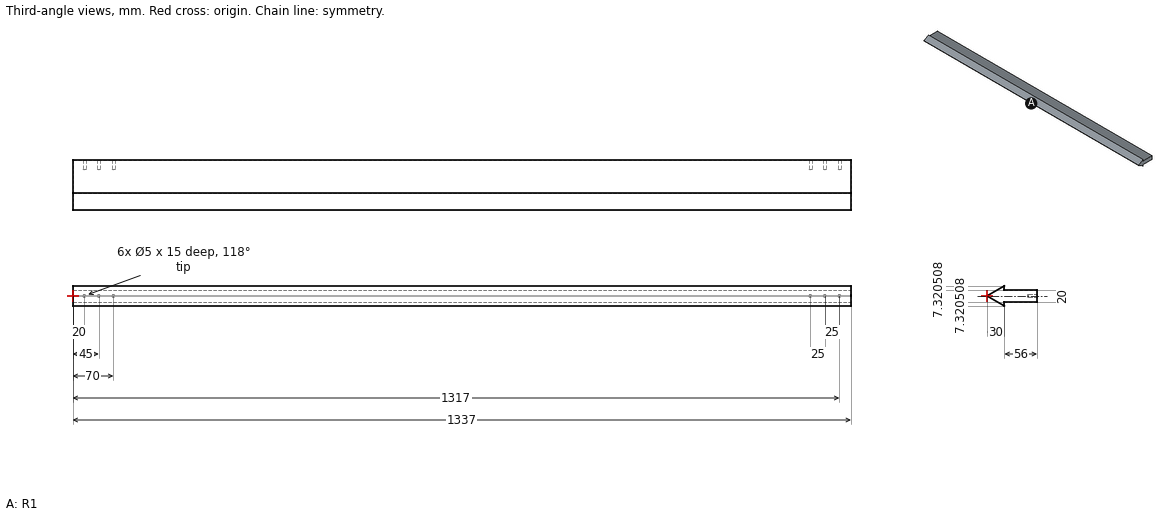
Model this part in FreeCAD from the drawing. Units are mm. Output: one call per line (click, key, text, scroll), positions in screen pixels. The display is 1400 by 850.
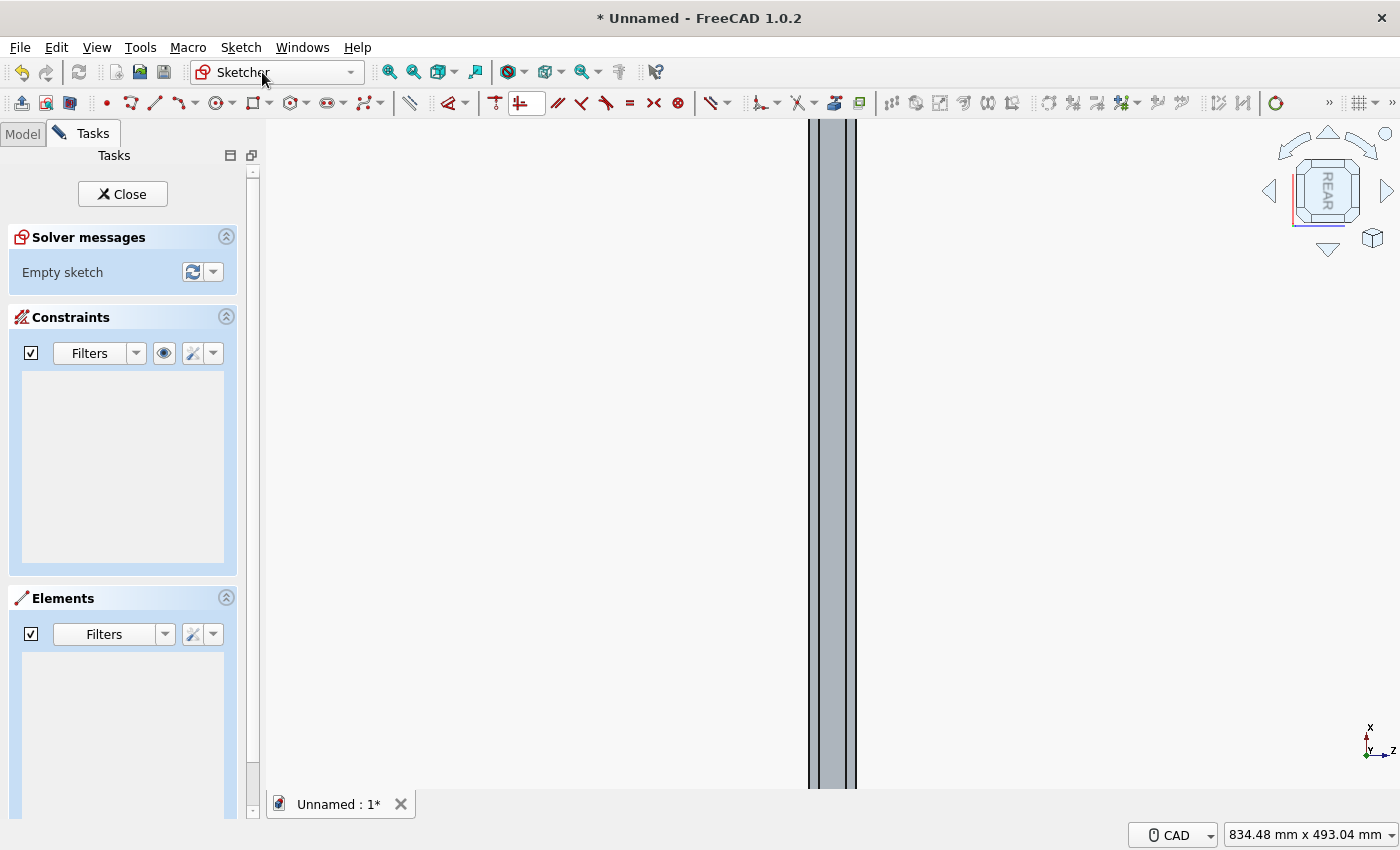
scroll(742, 450, down, 7)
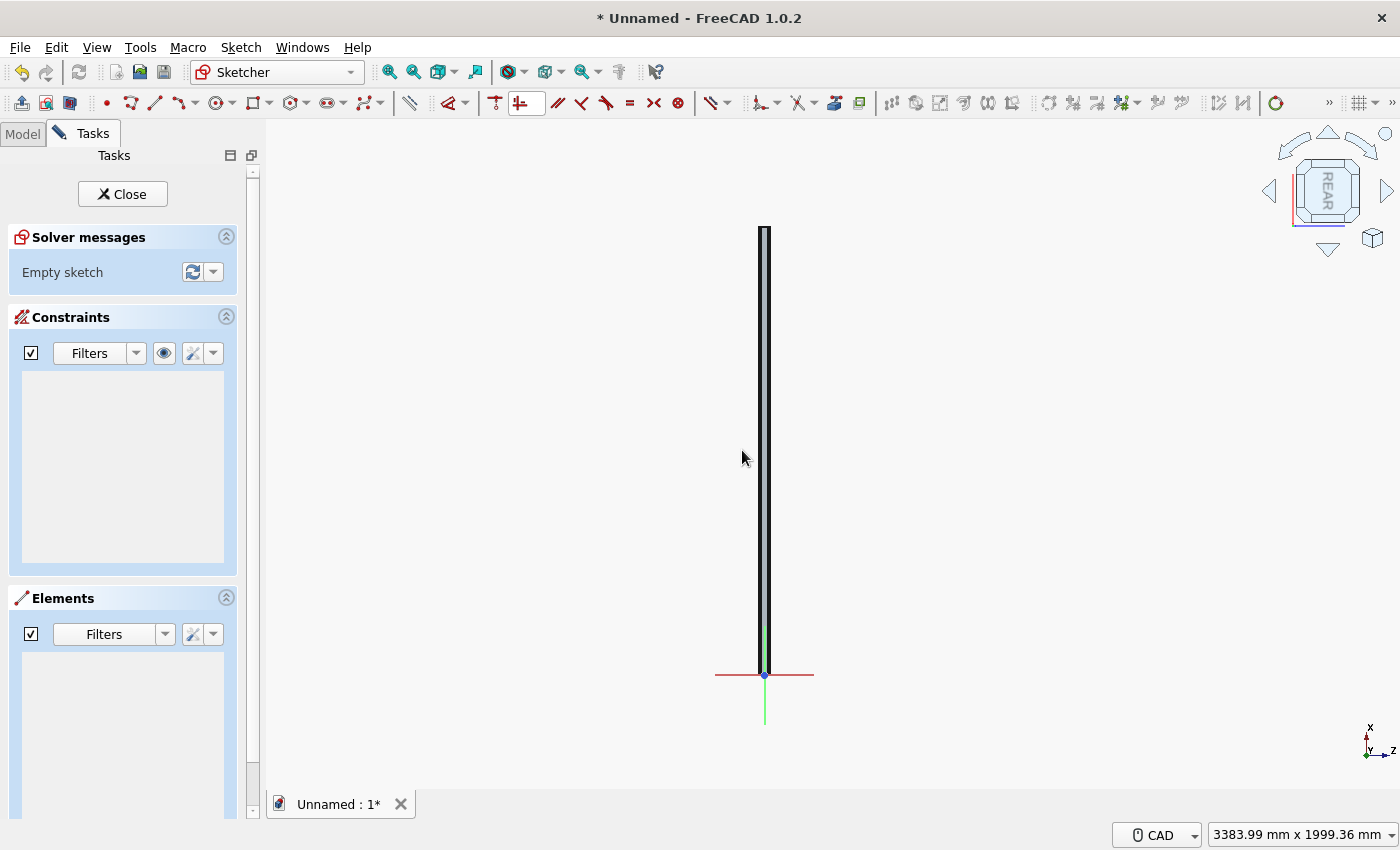
click(216, 104)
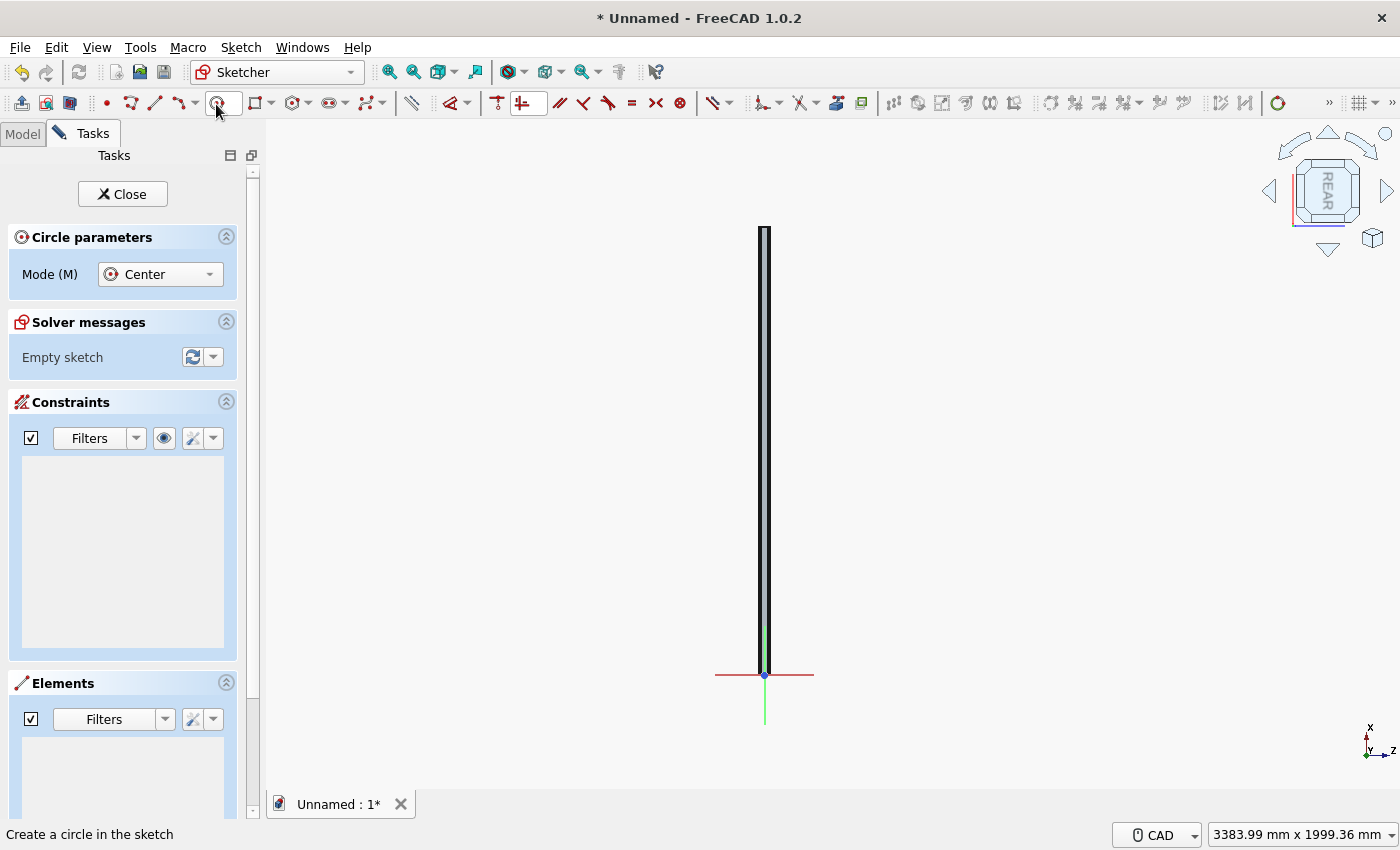
scroll(765, 668, up, 17)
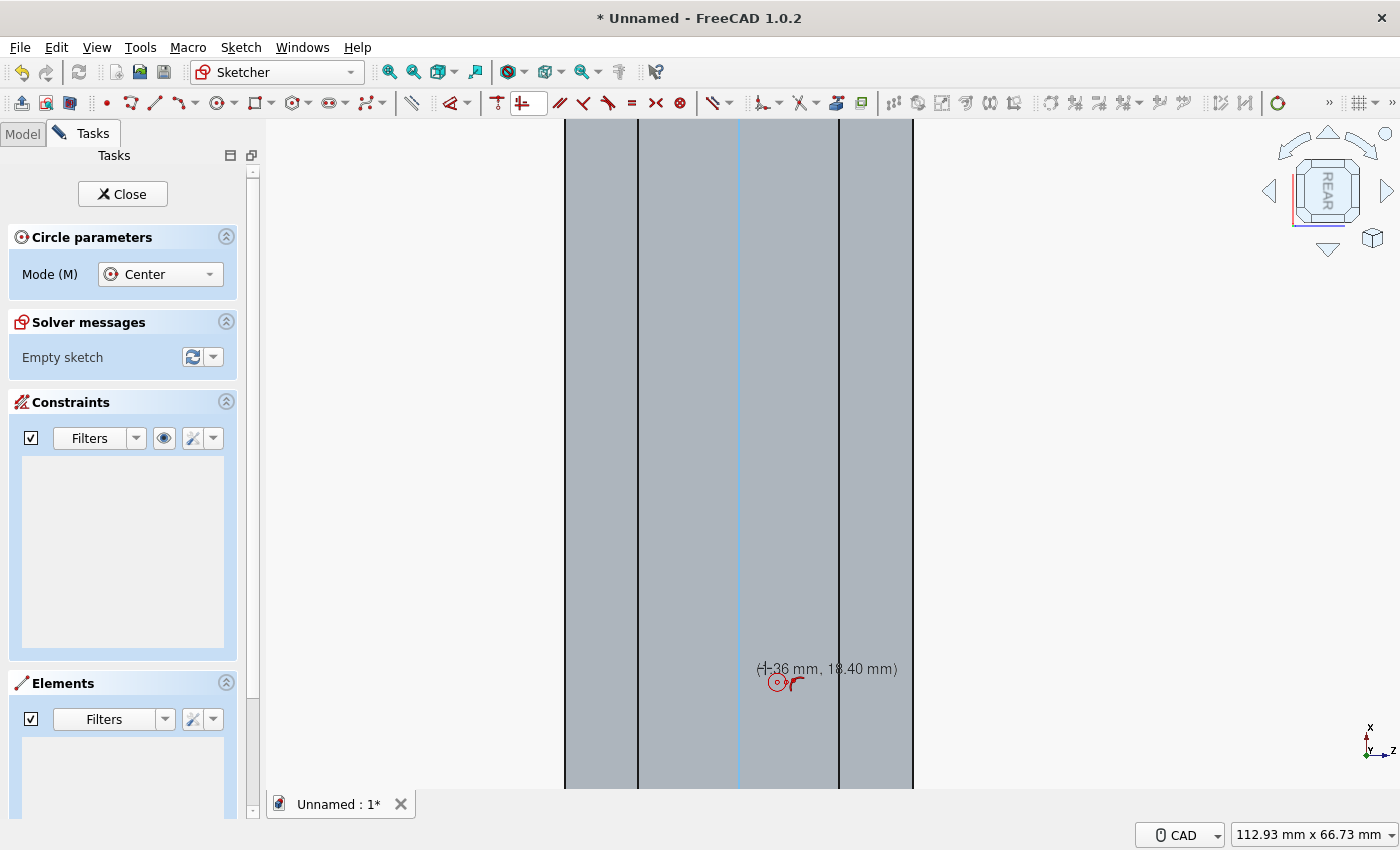
scroll(766, 718, down, 16)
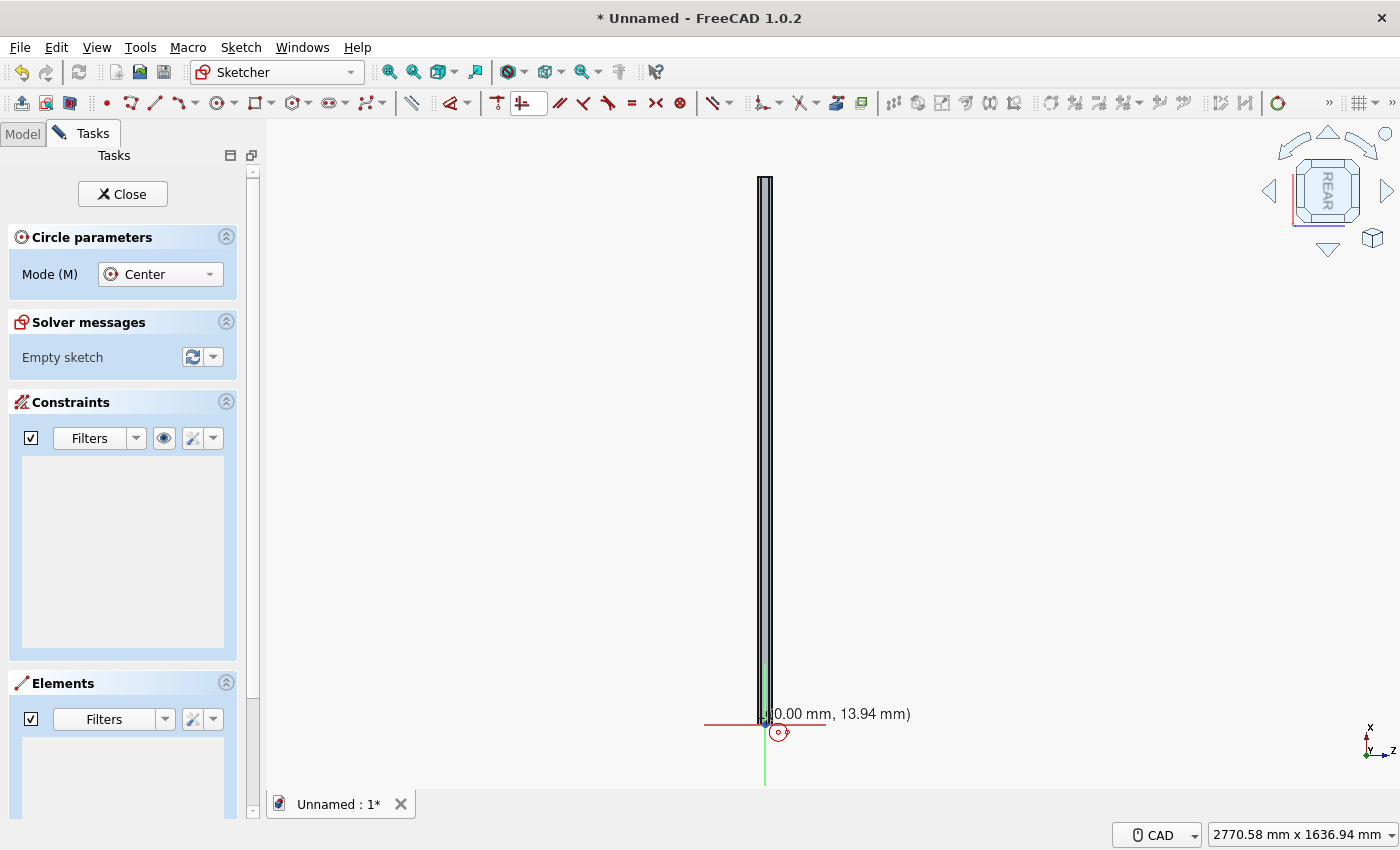
scroll(765, 716, up, 4)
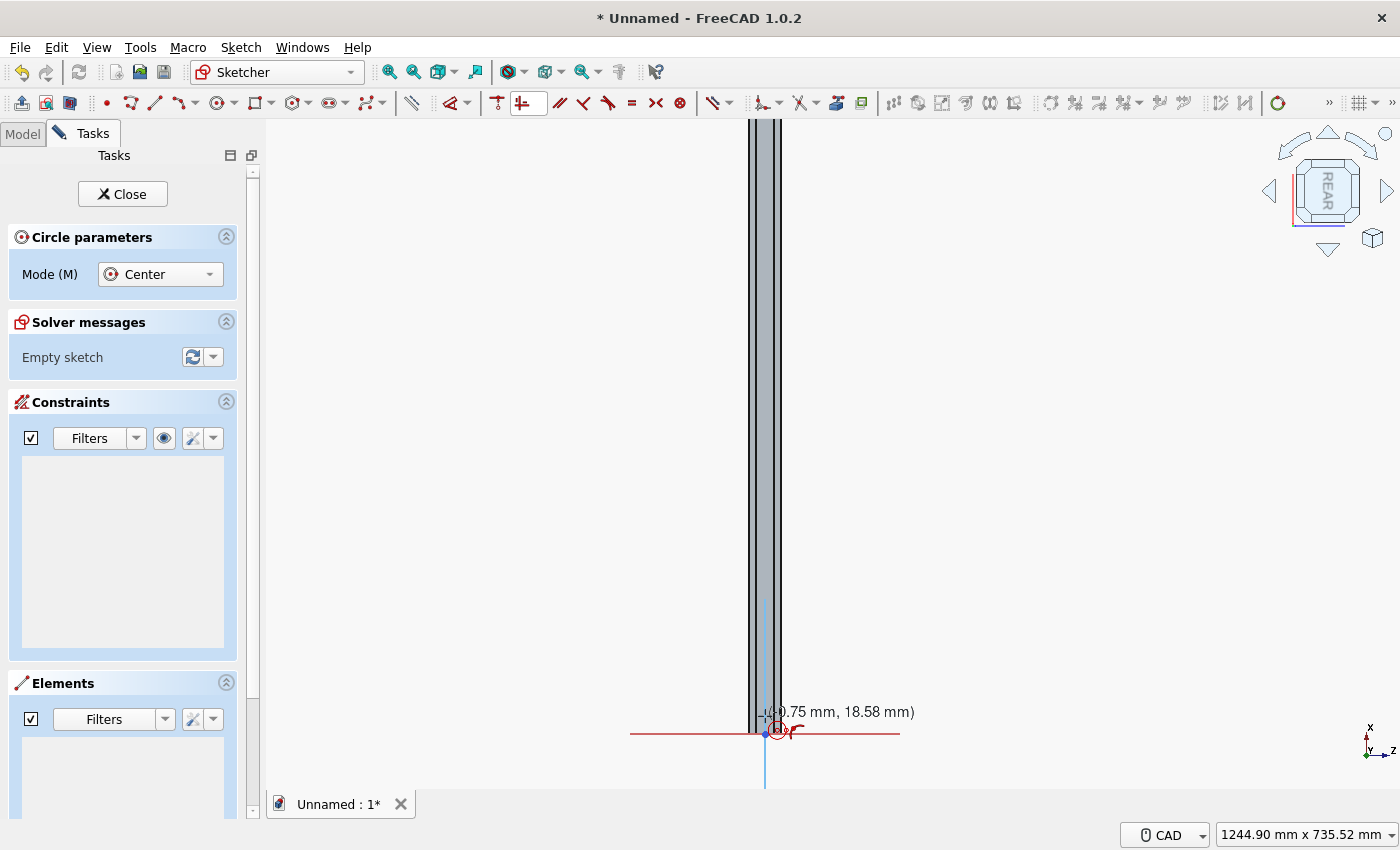
click(765, 716)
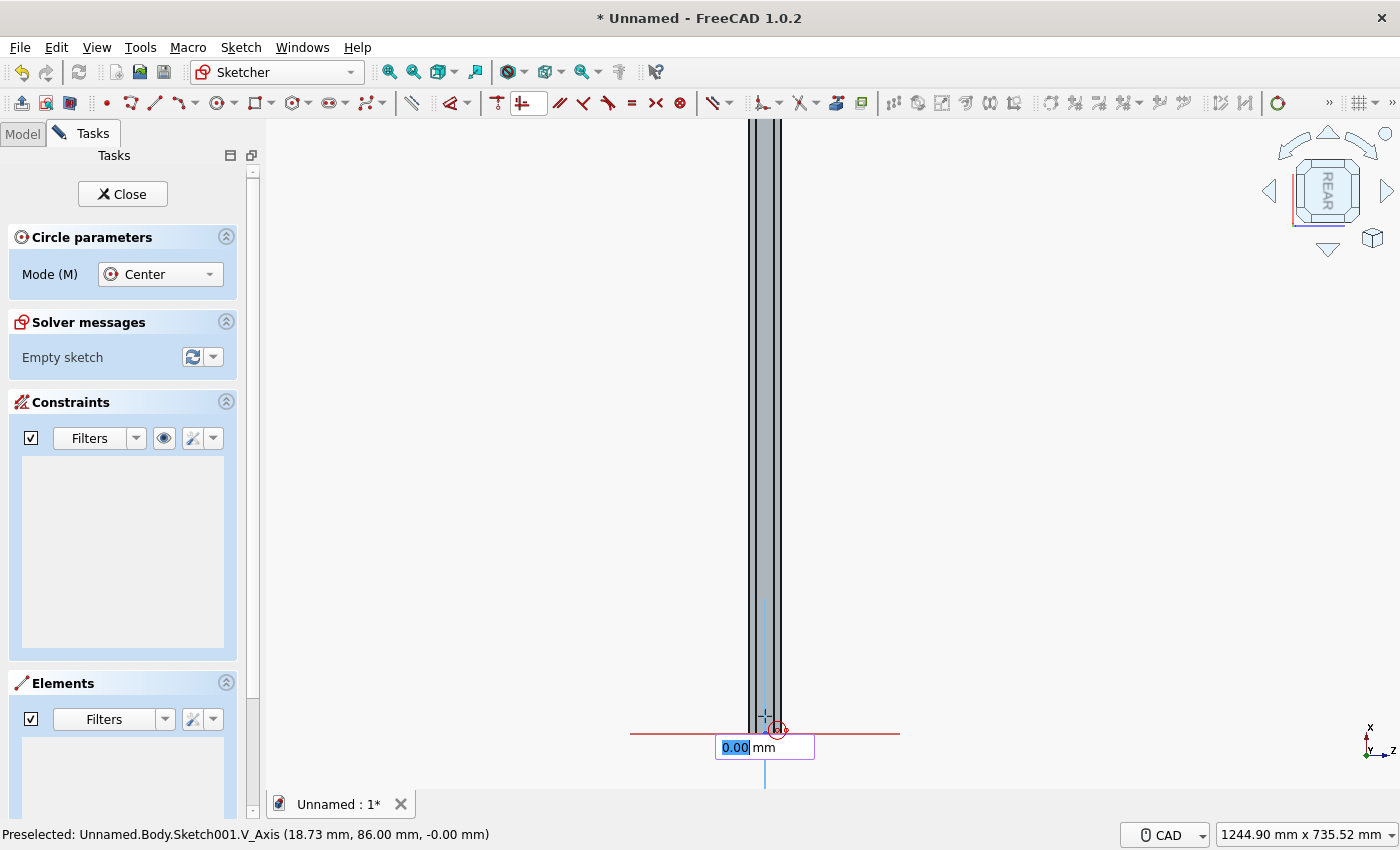
scroll(767, 715, up, 11)
move(766, 708)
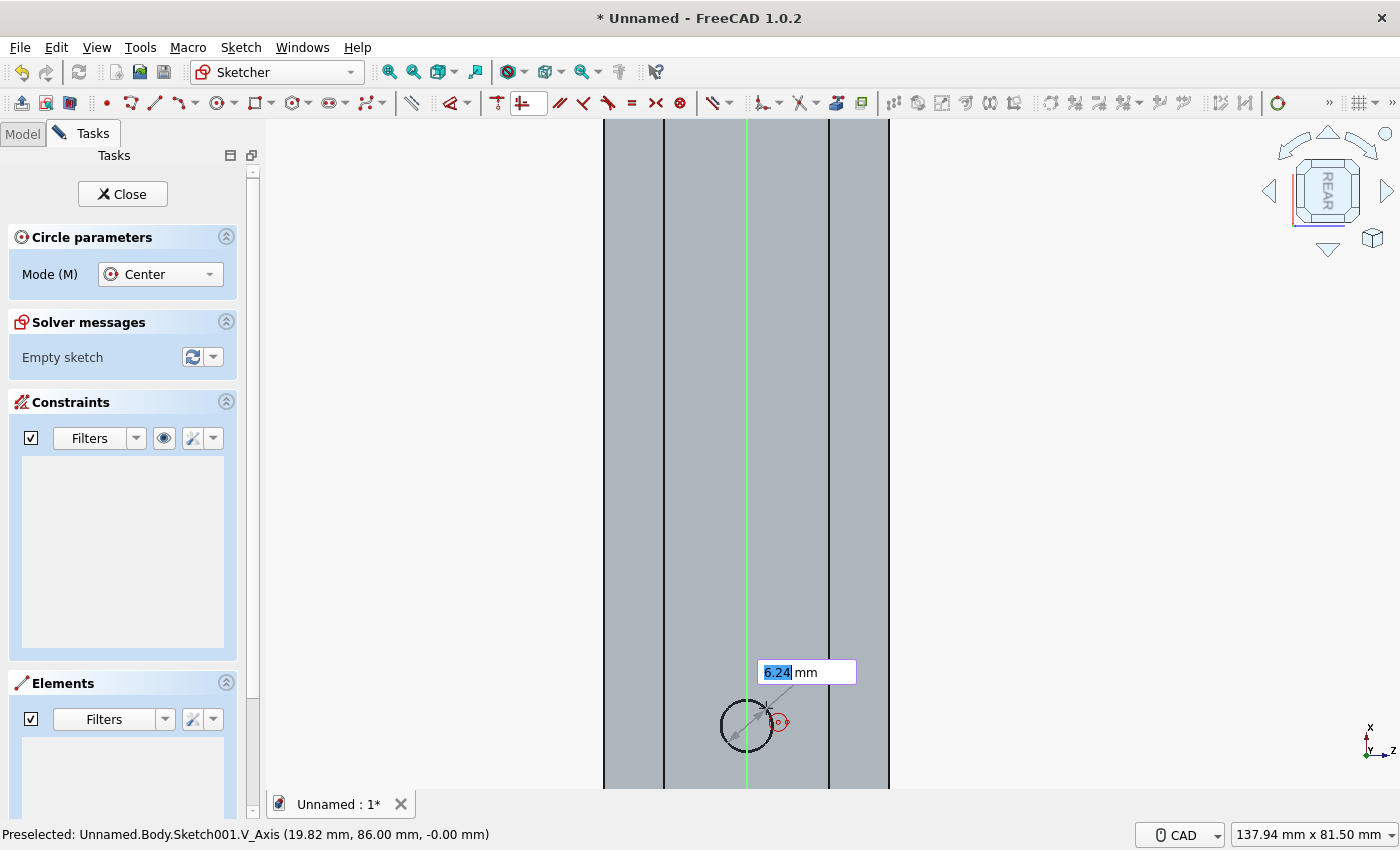
text(5)
key(Return)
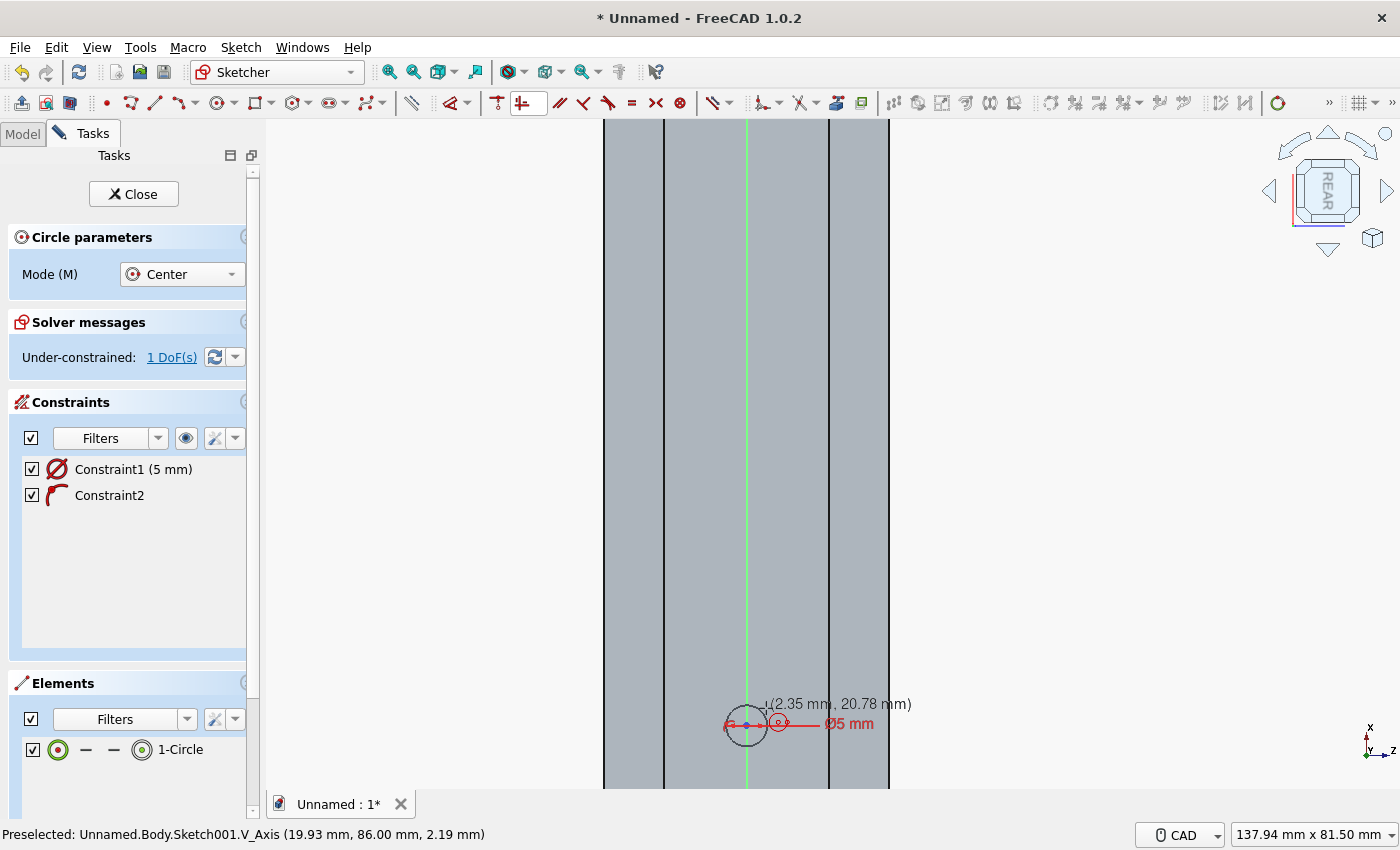
scroll(765, 716, down, 15)